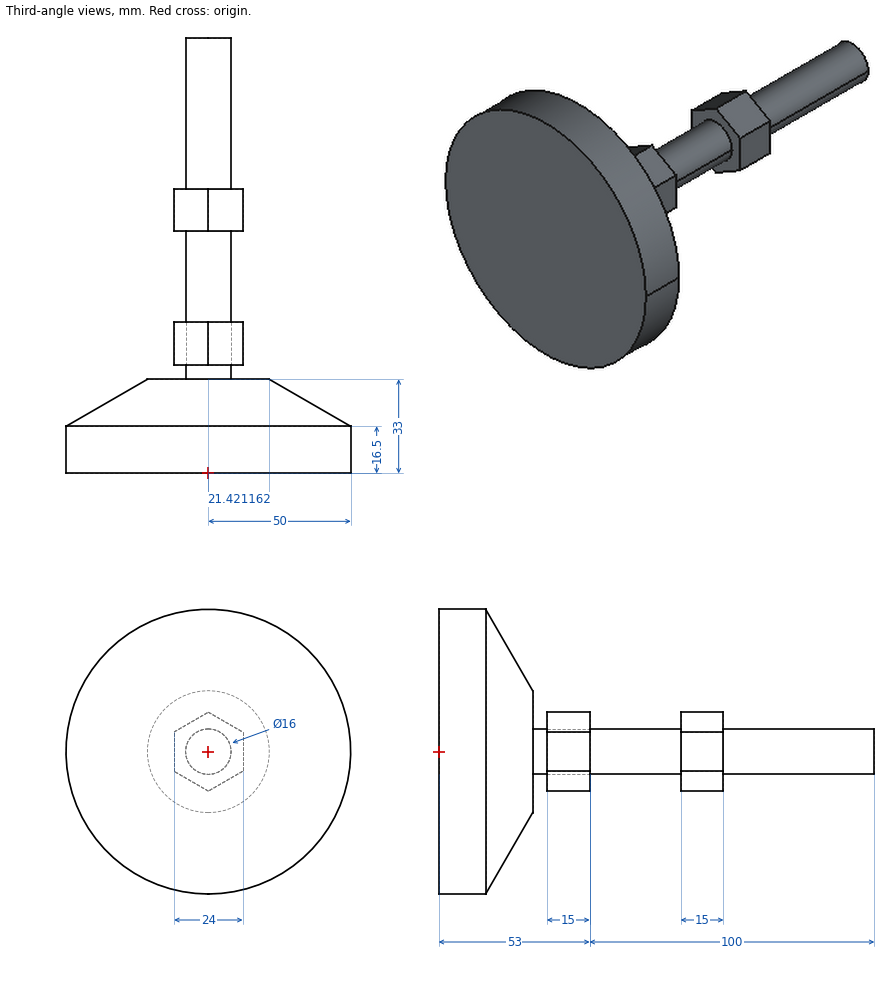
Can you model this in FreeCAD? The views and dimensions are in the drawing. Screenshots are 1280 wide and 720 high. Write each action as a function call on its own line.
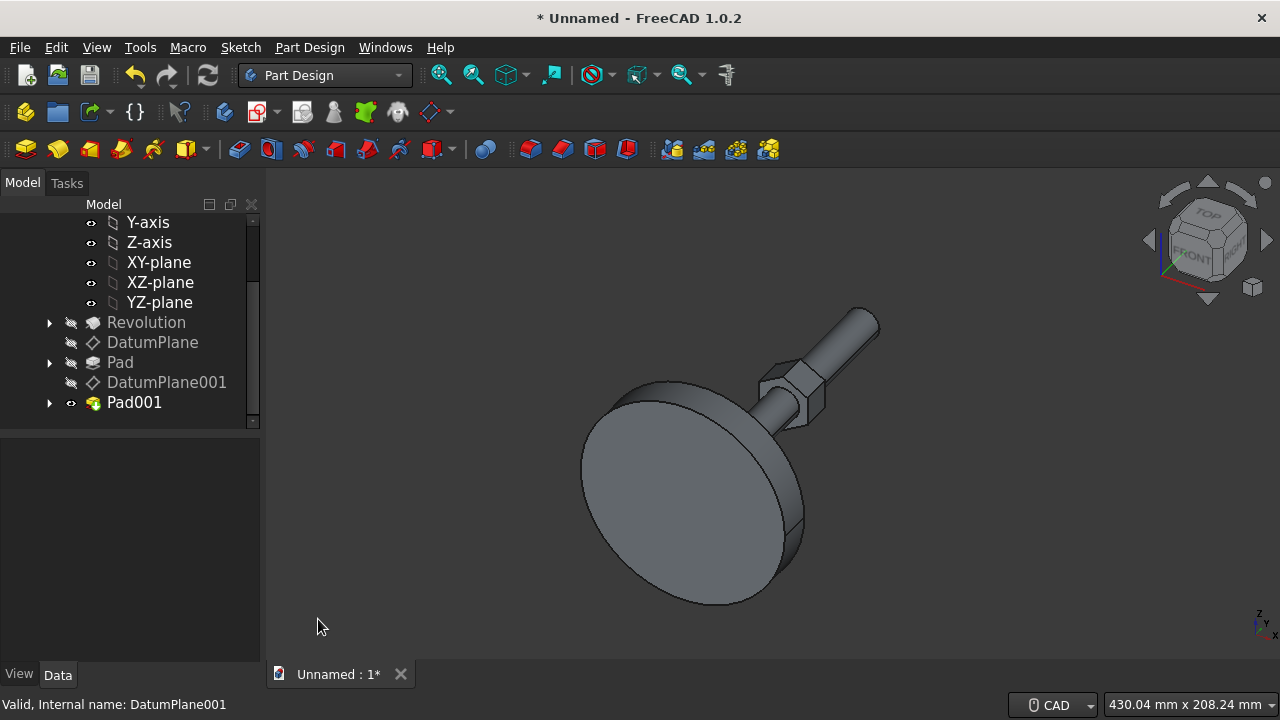
click(226, 112)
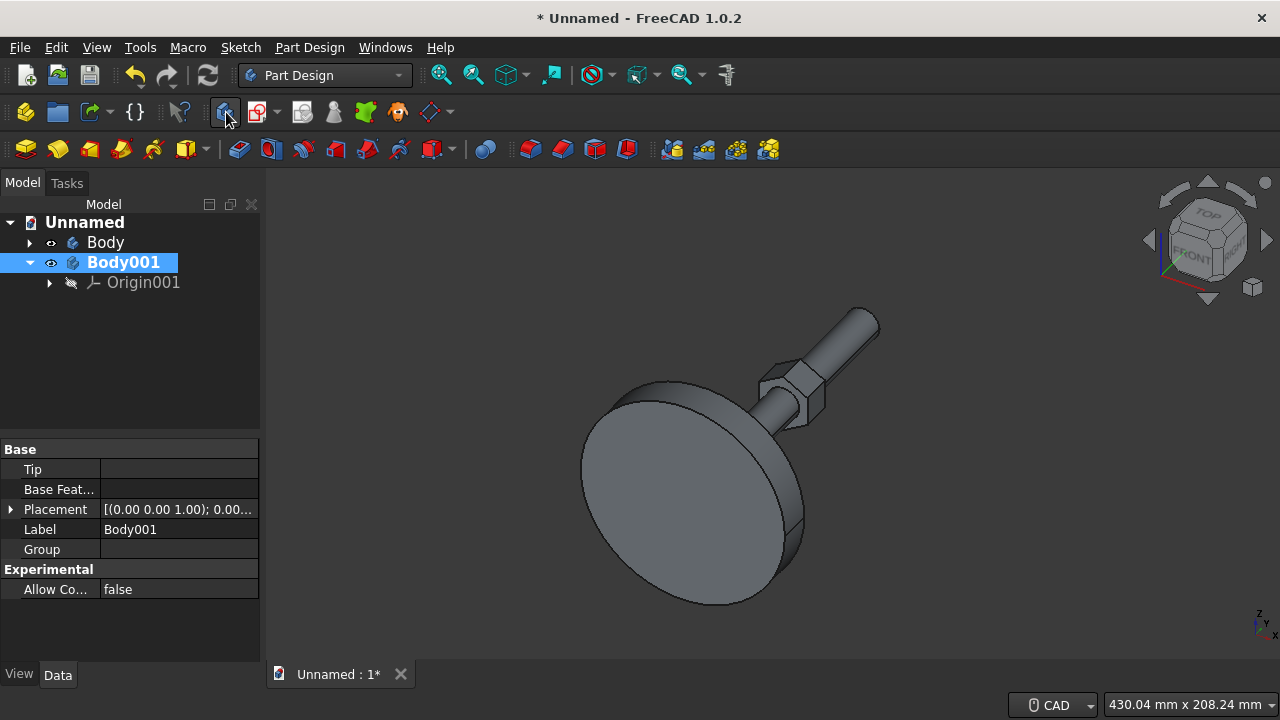
click(50, 283)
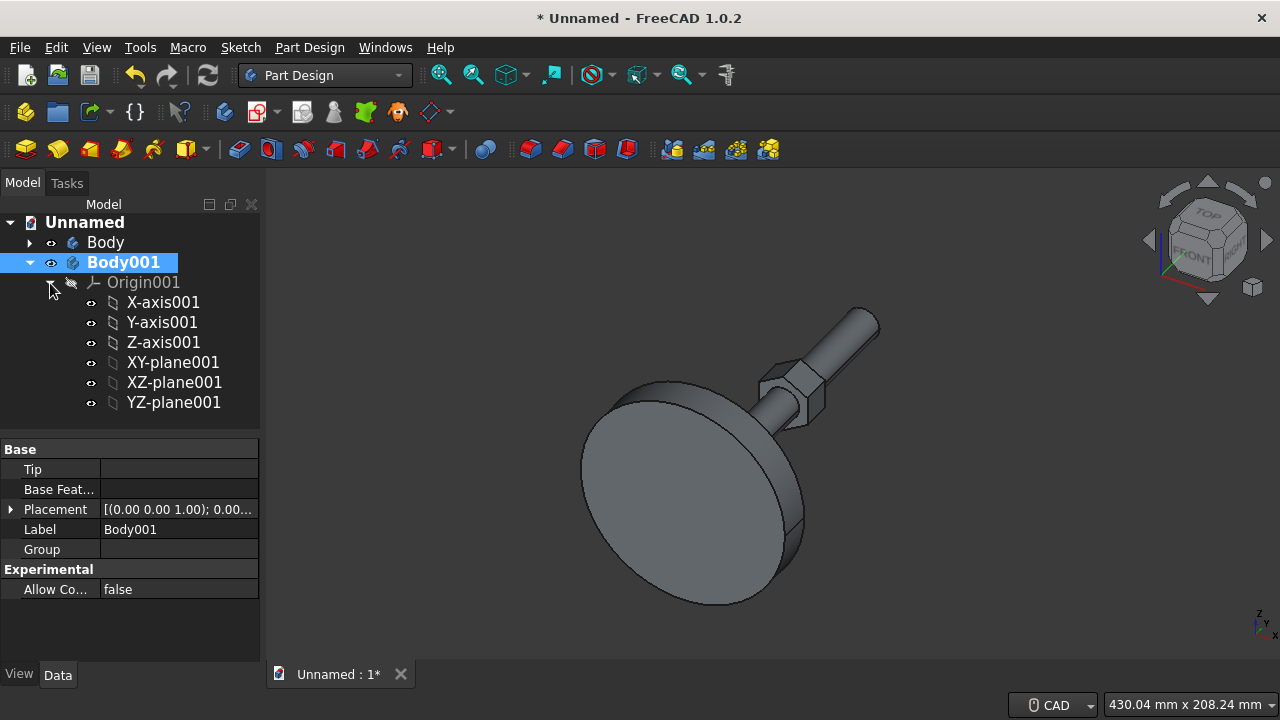
click(136, 383)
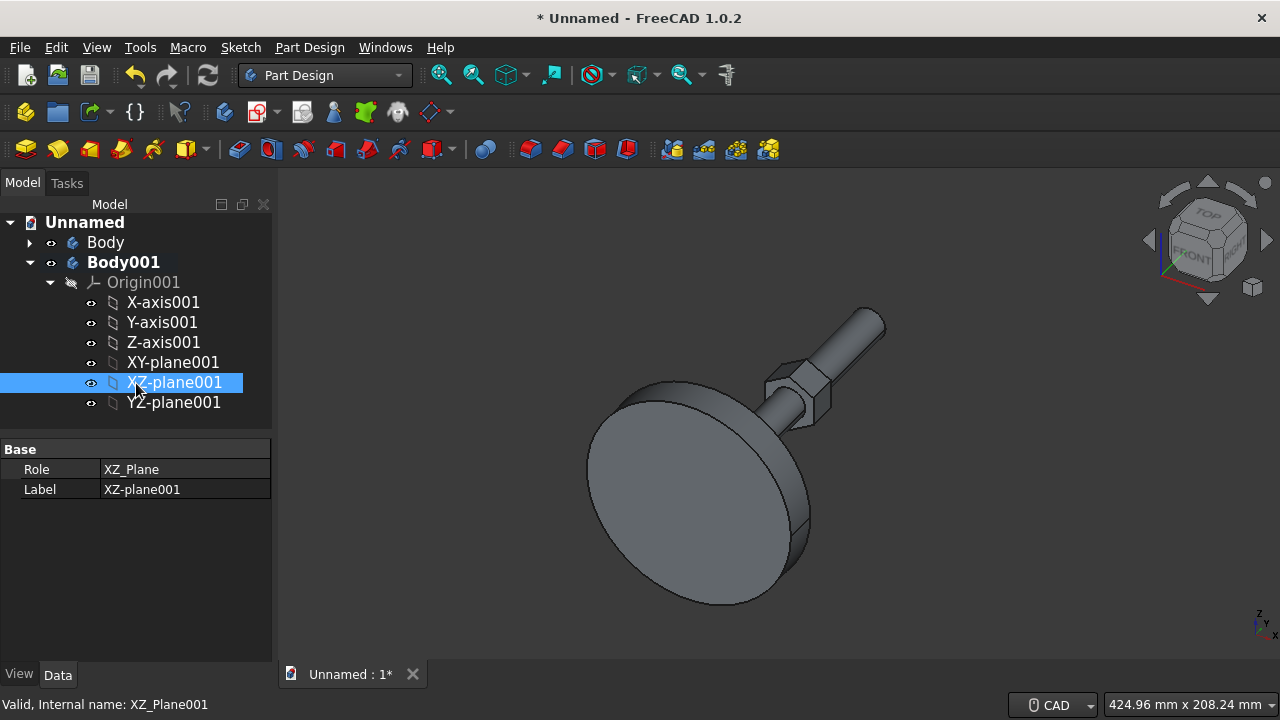
click(430, 112)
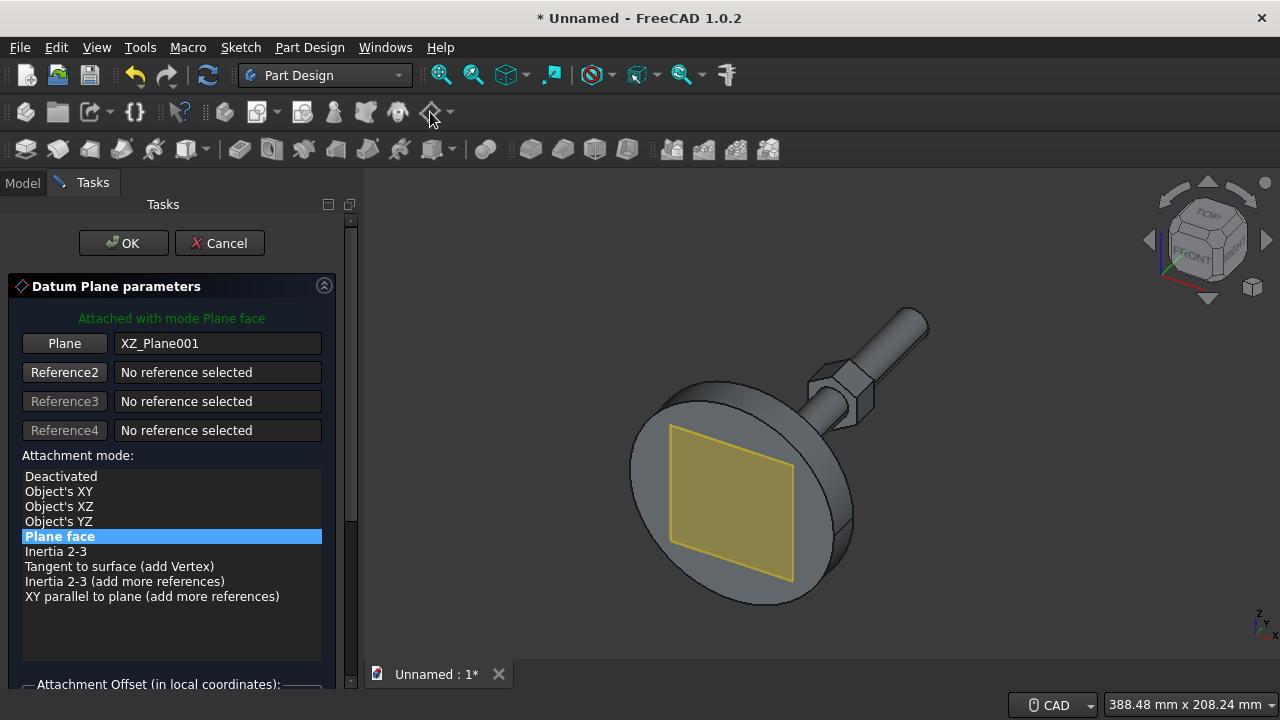
scroll(351, 451, down, 3)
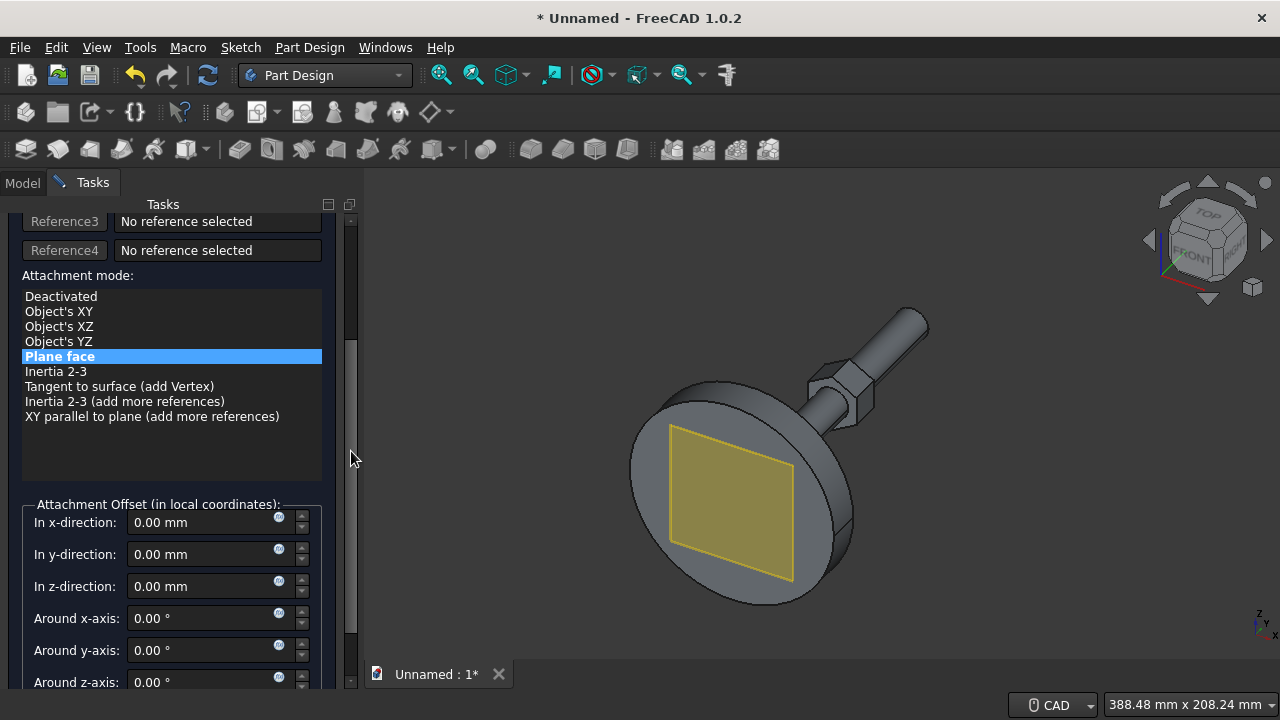
triple_click(210, 586)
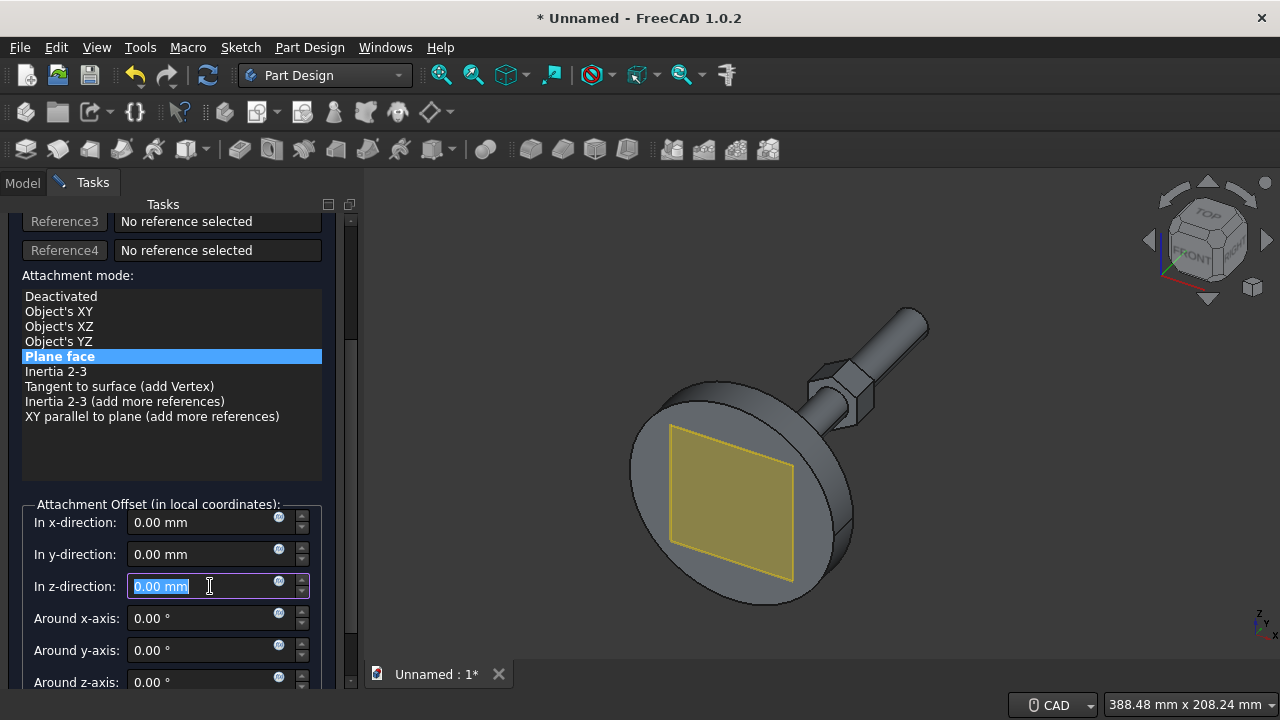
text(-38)
key(Tab)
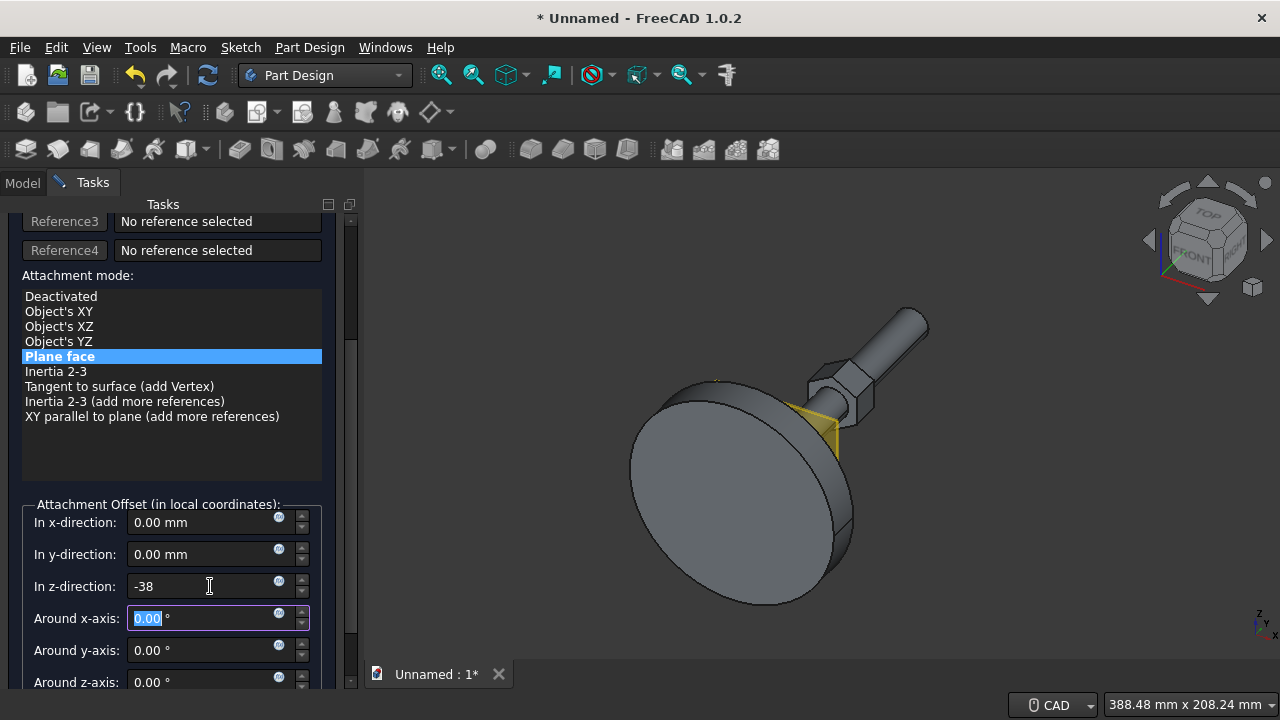
scroll(351, 451, up, 4)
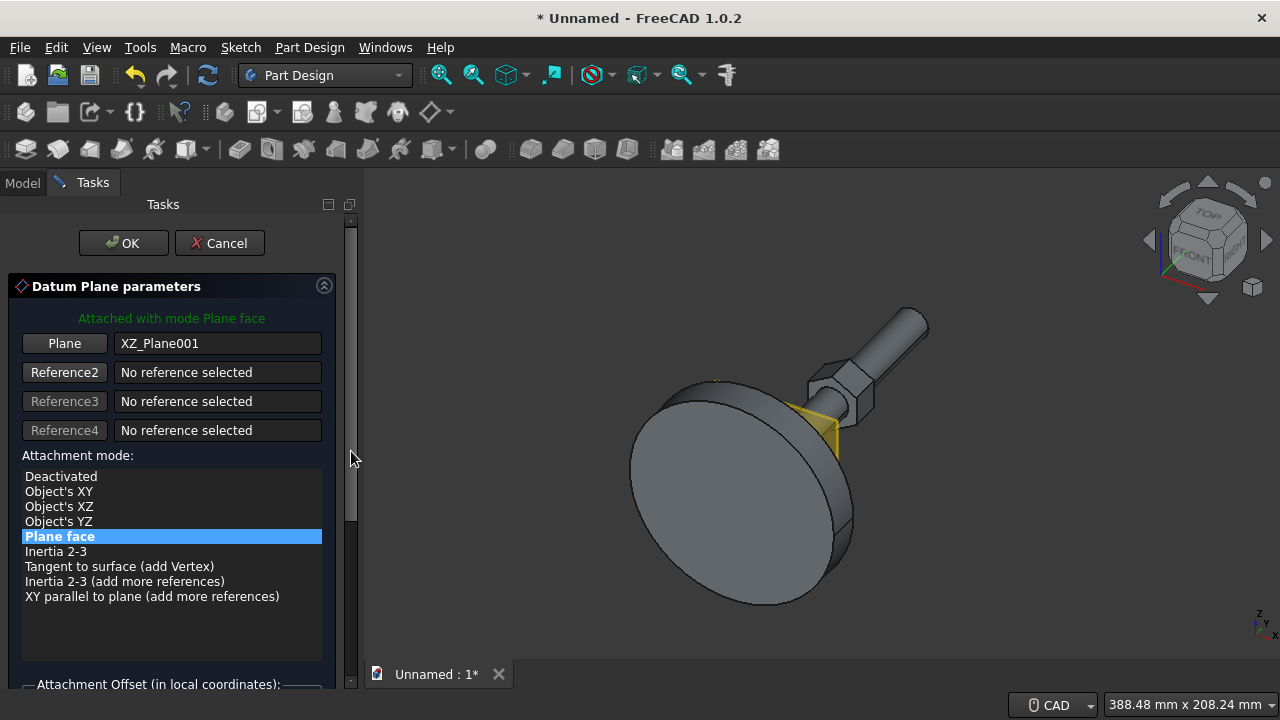
click(124, 243)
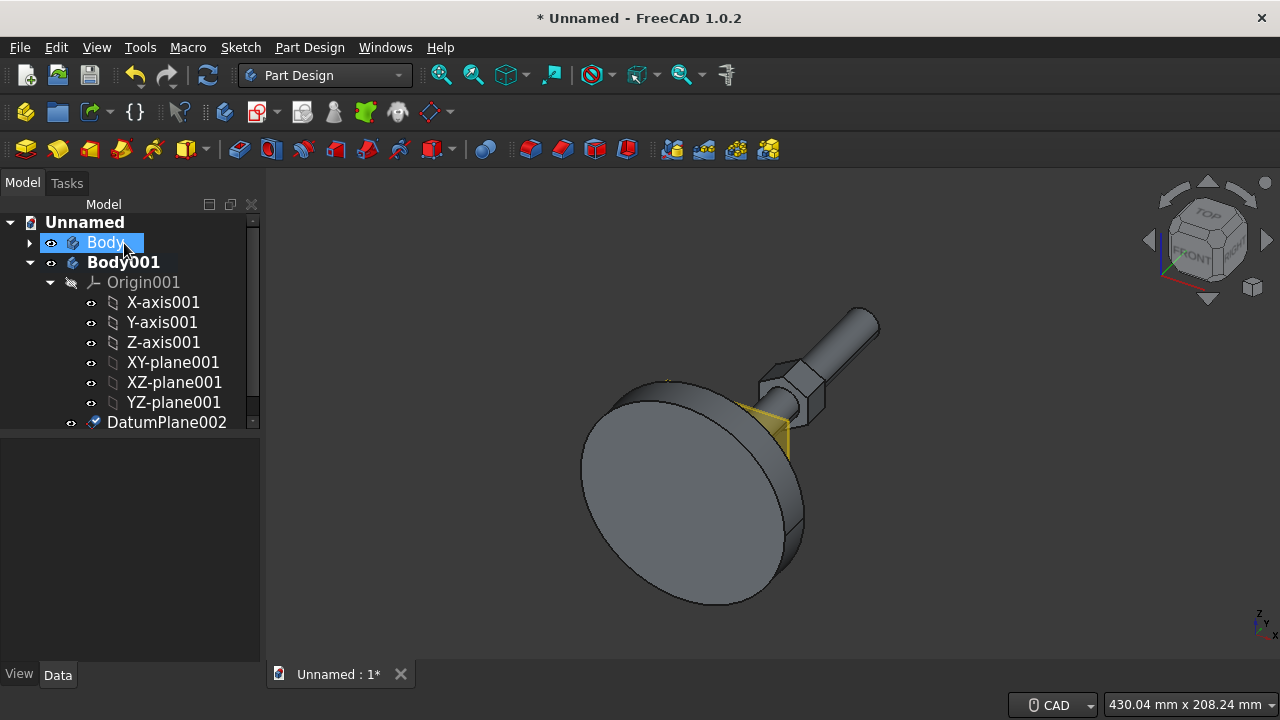
click(116, 423)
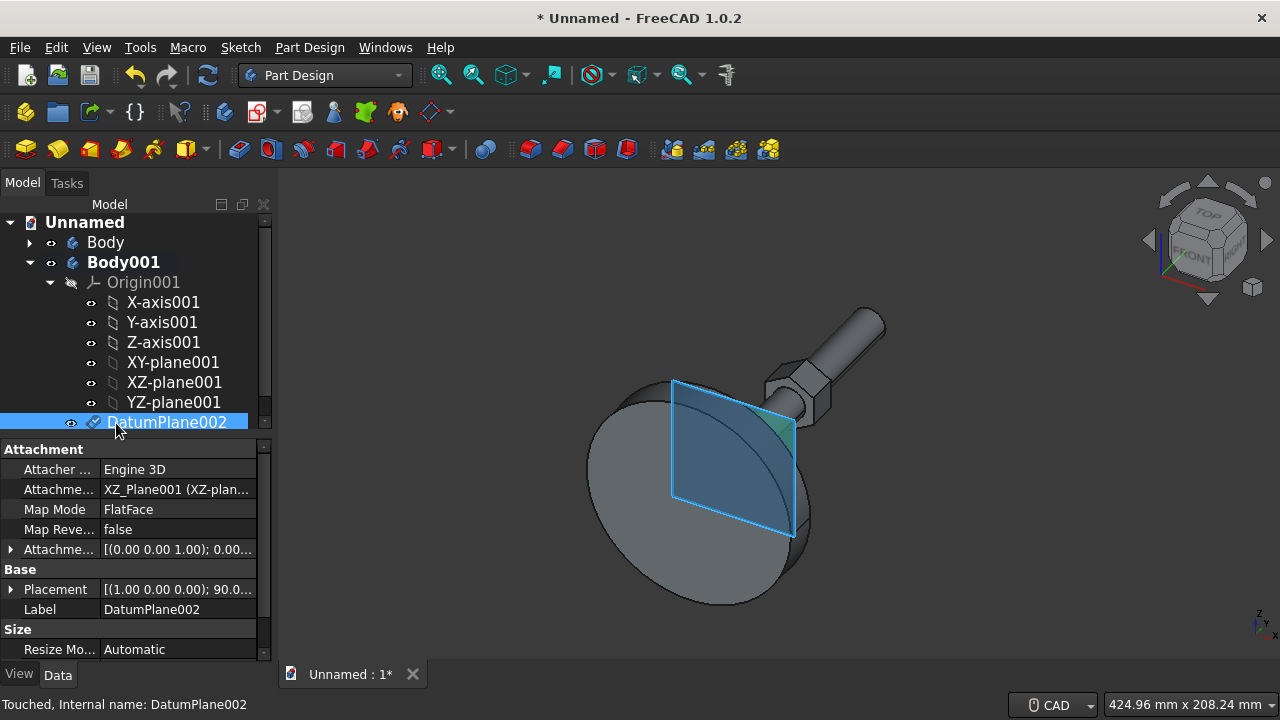
click(258, 112)